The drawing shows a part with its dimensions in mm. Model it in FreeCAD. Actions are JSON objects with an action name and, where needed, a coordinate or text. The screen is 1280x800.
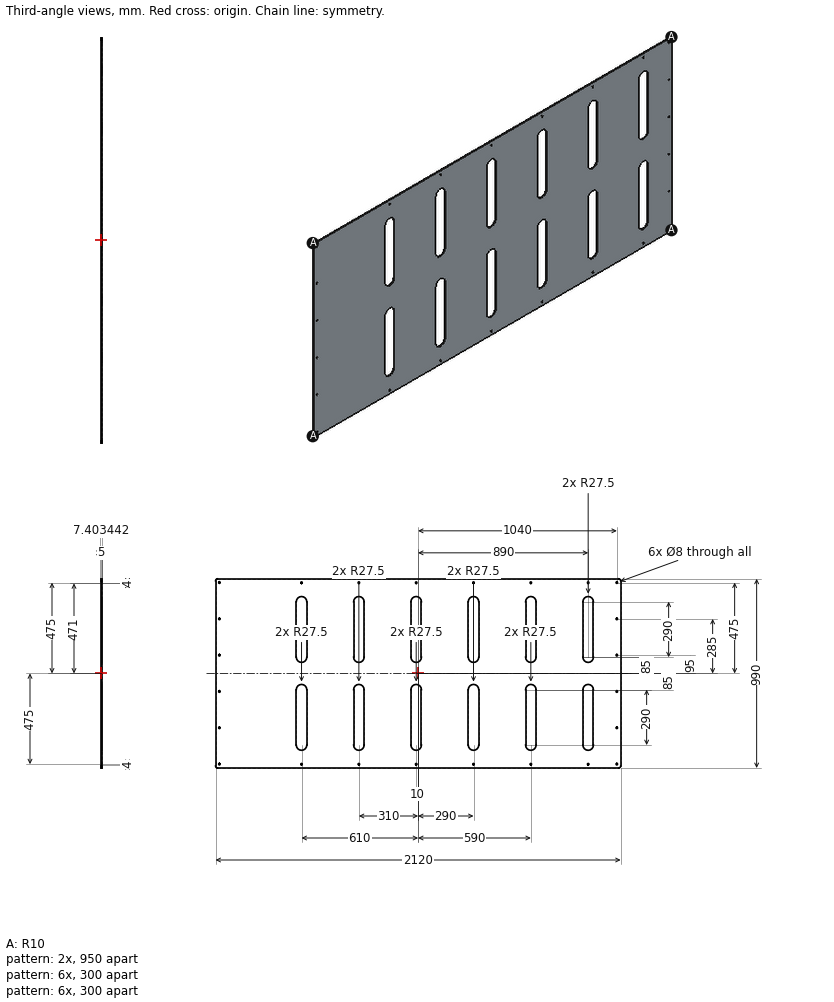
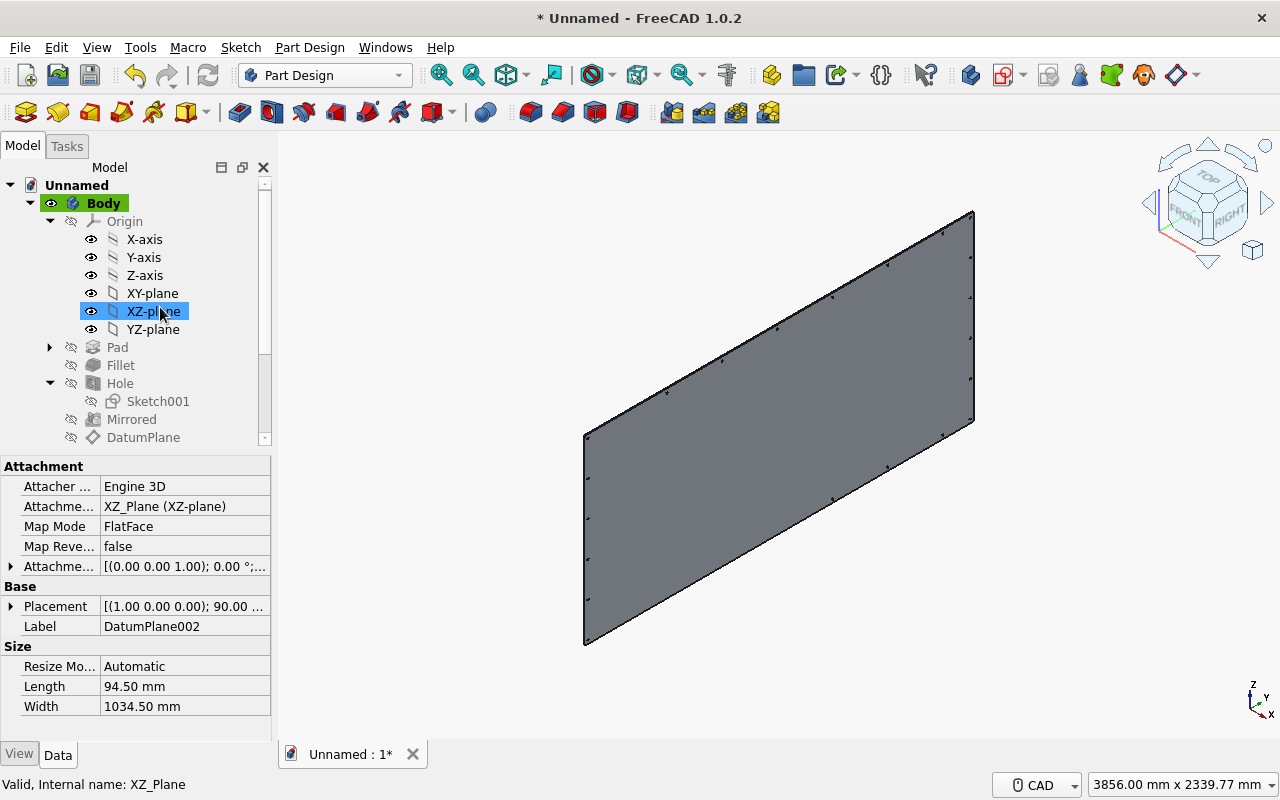
{"action": "left_click", "coordinate": [136, 311]}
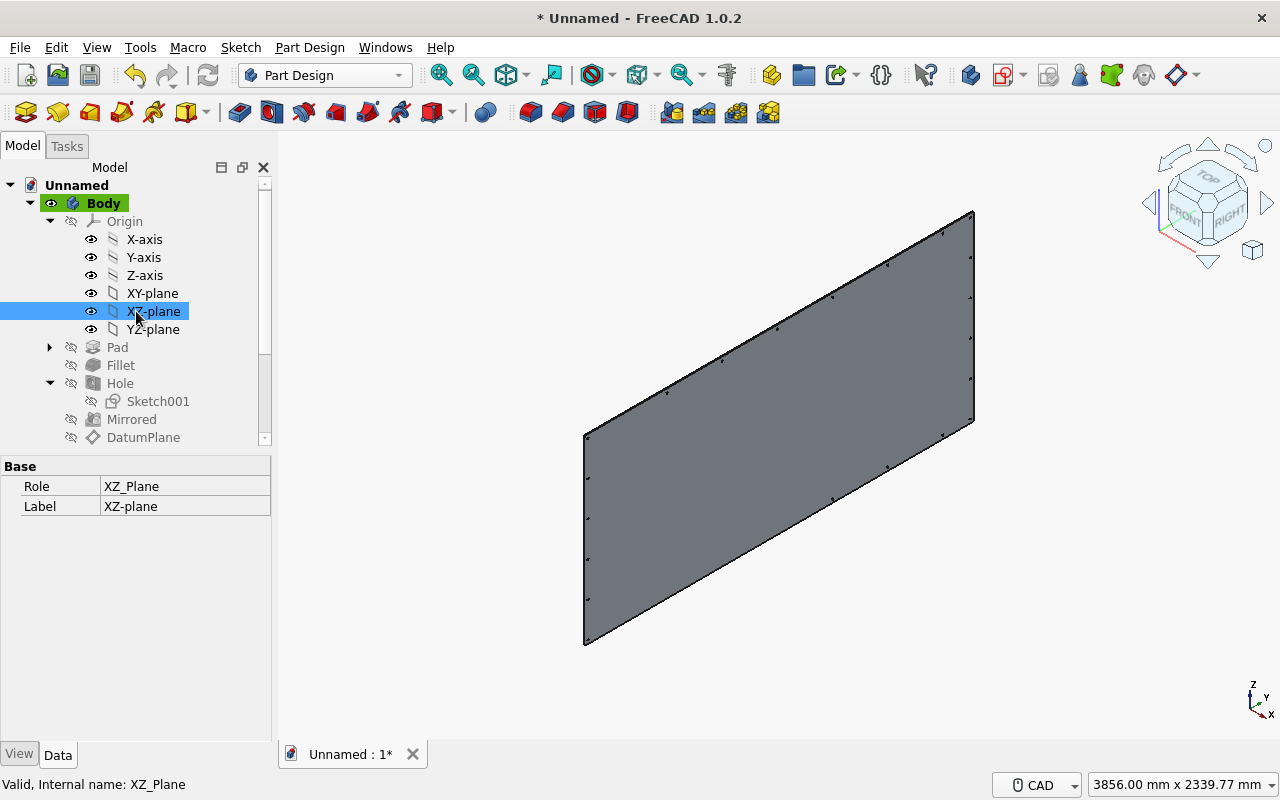
{"action": "left_click", "coordinate": [1176, 76]}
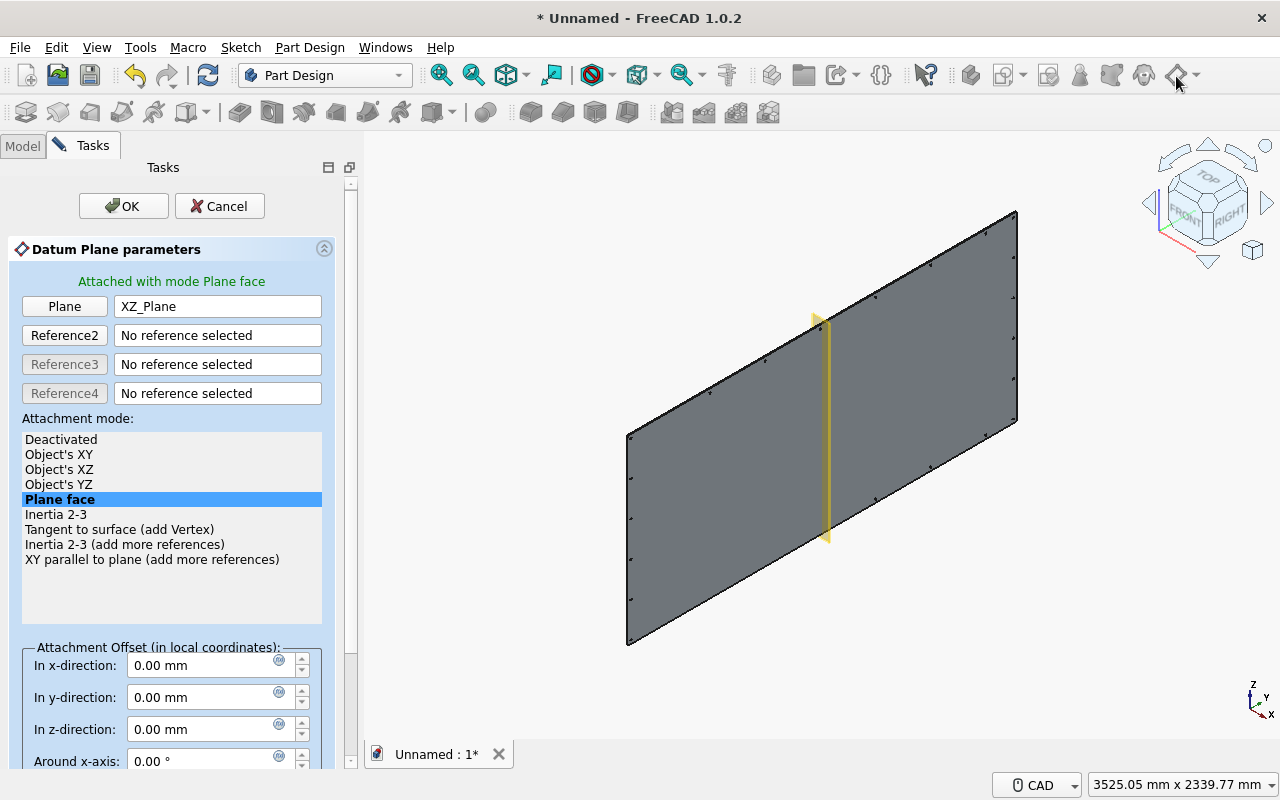
{"action": "triple_click", "coordinate": [210, 729]}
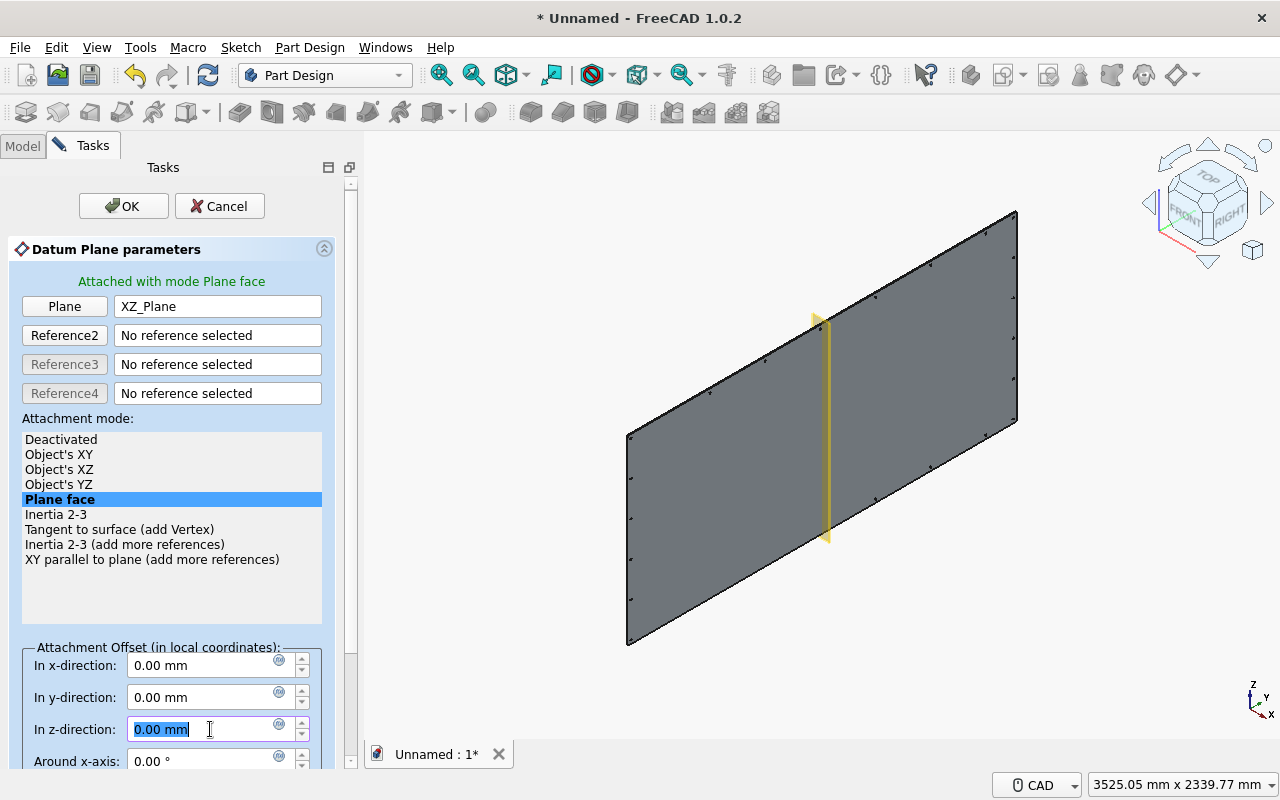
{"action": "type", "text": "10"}
{"action": "key", "text": "Tab"}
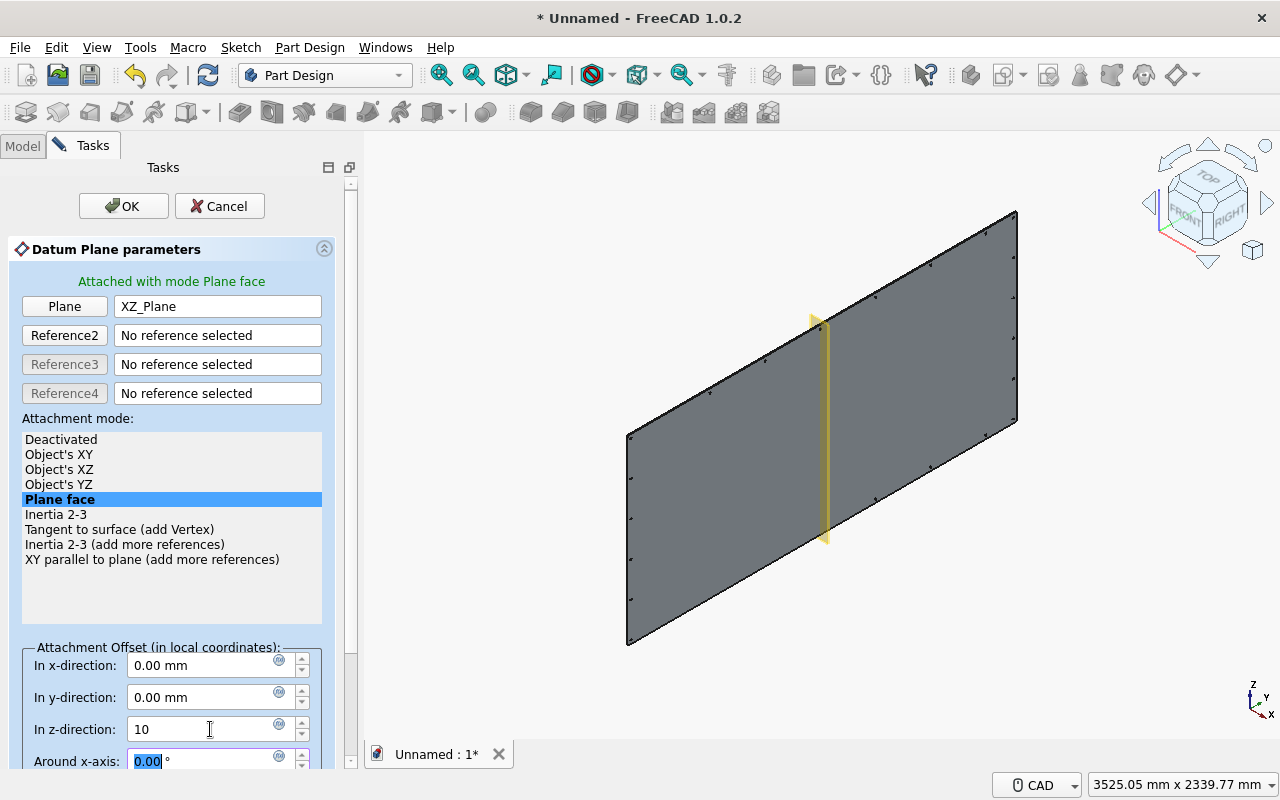
{"action": "left_click", "coordinate": [124, 206]}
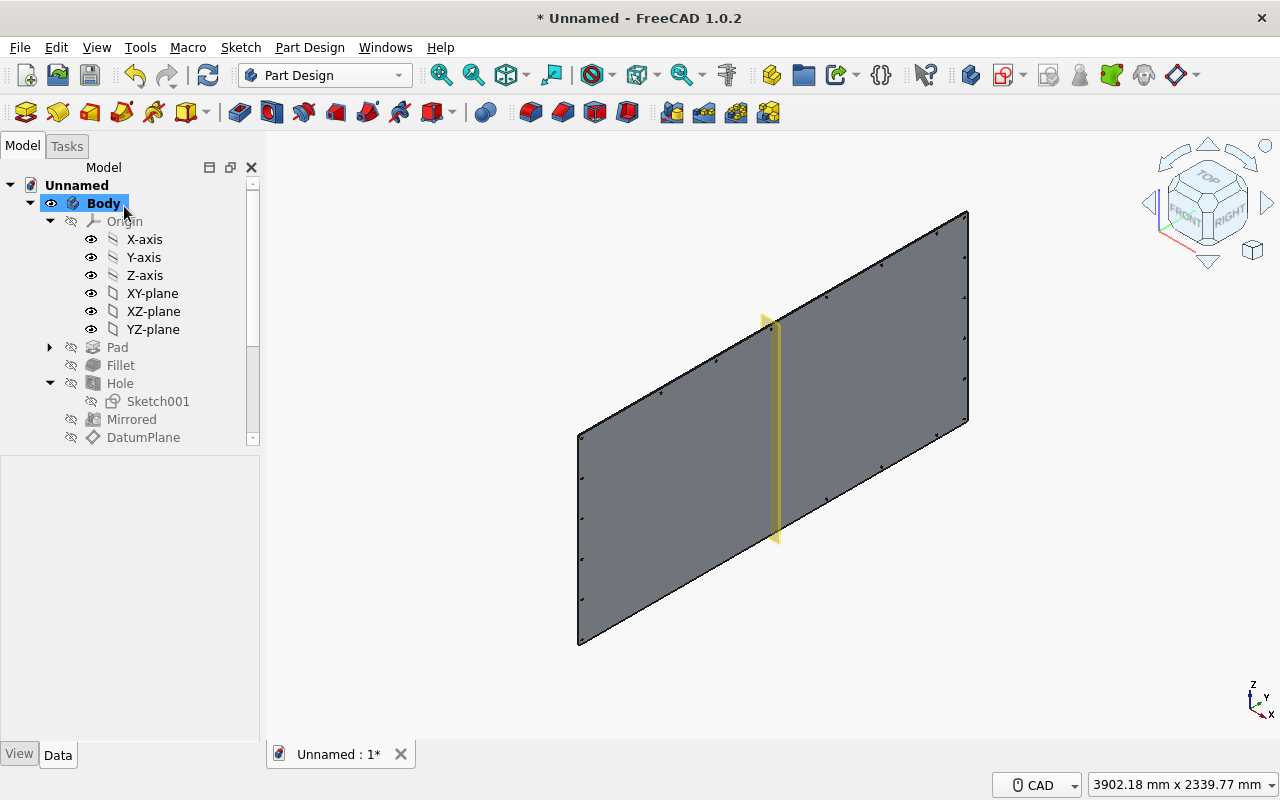
{"action": "scroll", "coordinate": [100, 307], "scroll_direction": "down", "scroll_amount": 3}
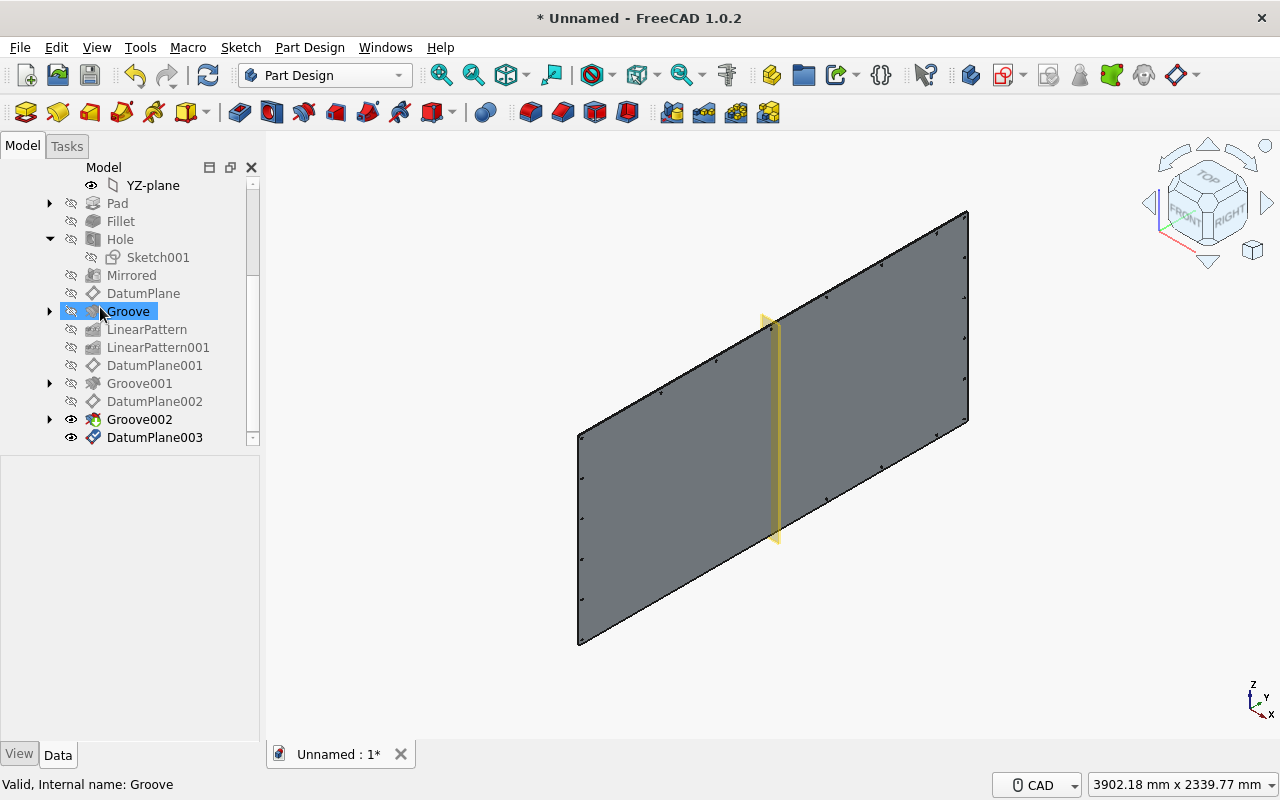
{"action": "left_click", "coordinate": [116, 437]}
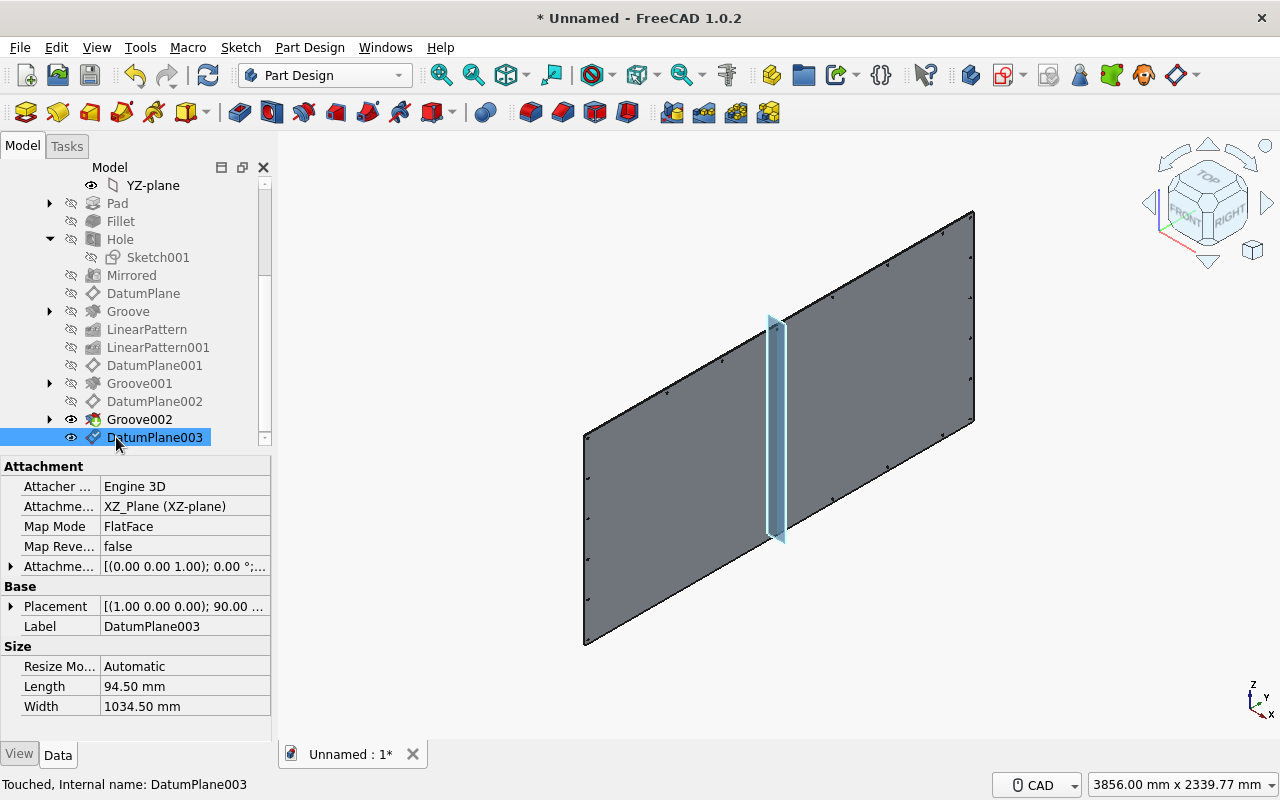
{"action": "left_click", "coordinate": [1004, 76]}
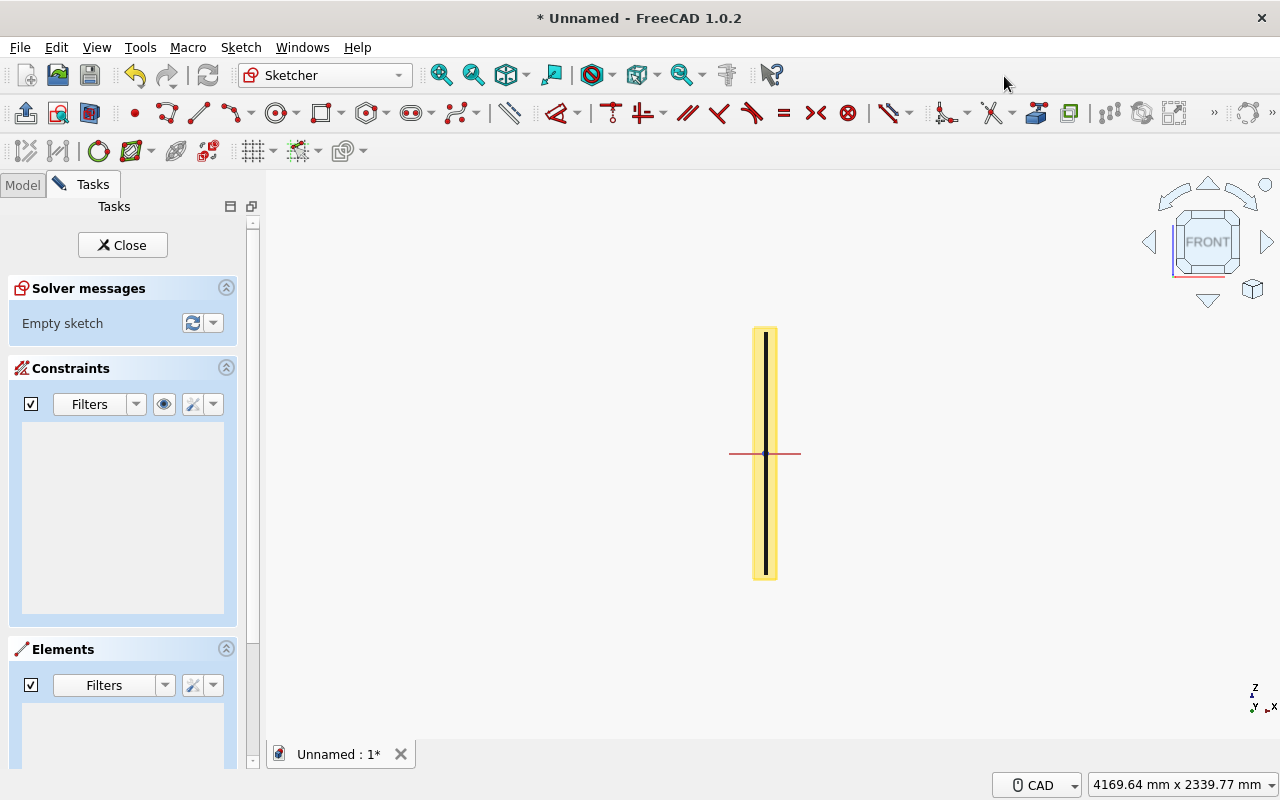
{"action": "left_click", "coordinate": [90, 114]}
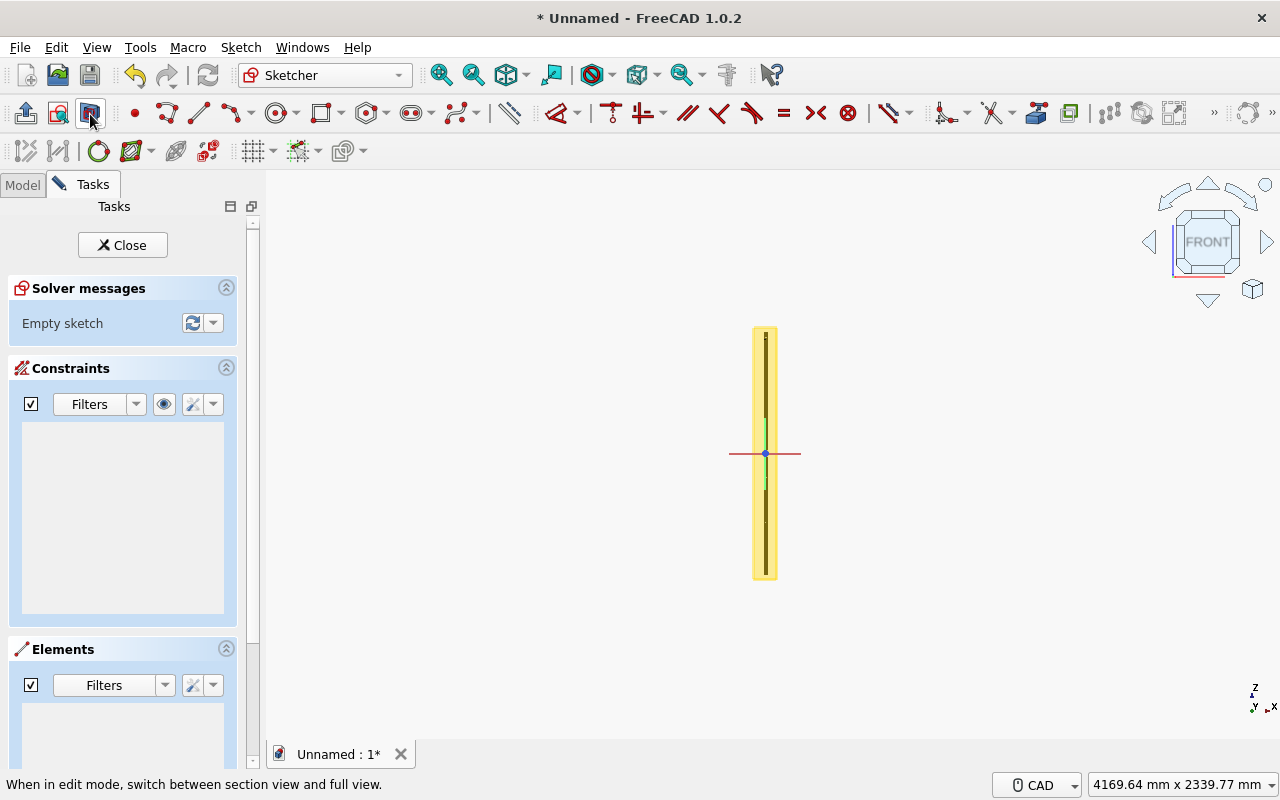
{"action": "scroll", "coordinate": [769, 576], "scroll_direction": "up", "scroll_amount": 15}